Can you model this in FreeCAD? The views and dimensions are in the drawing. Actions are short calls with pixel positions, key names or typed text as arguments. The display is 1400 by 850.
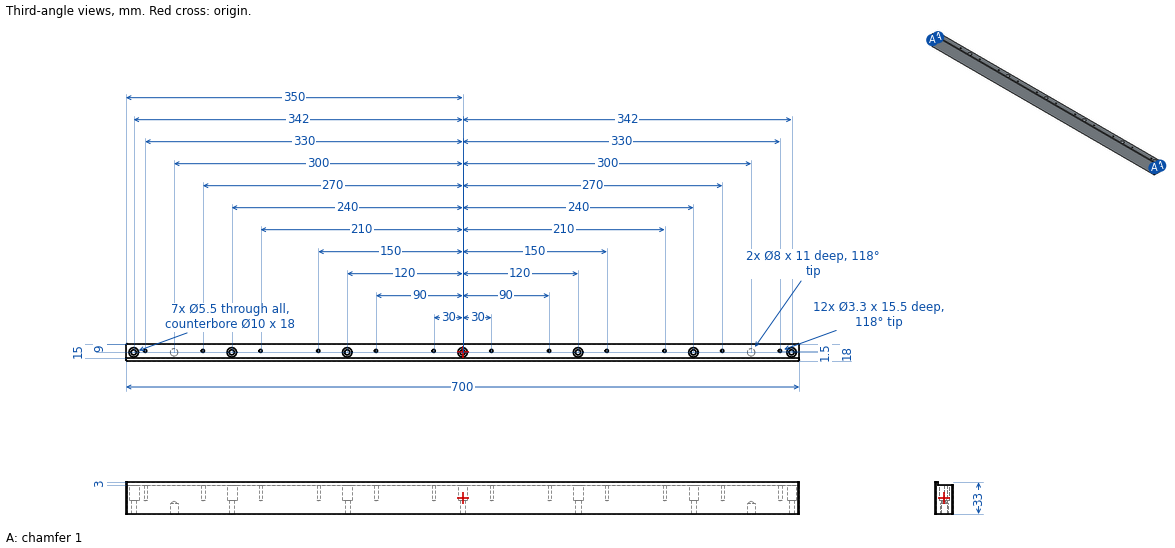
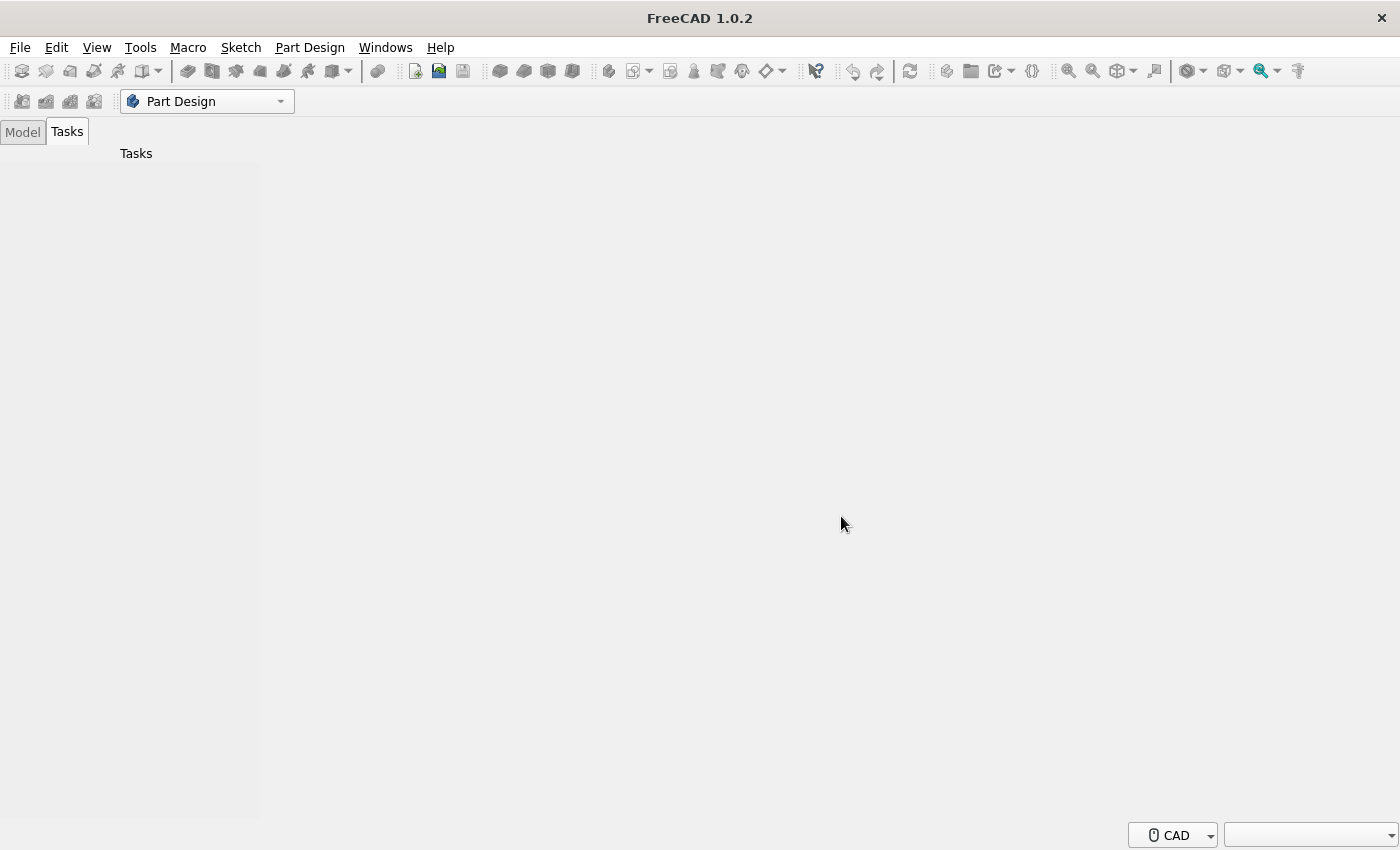
click(416, 72)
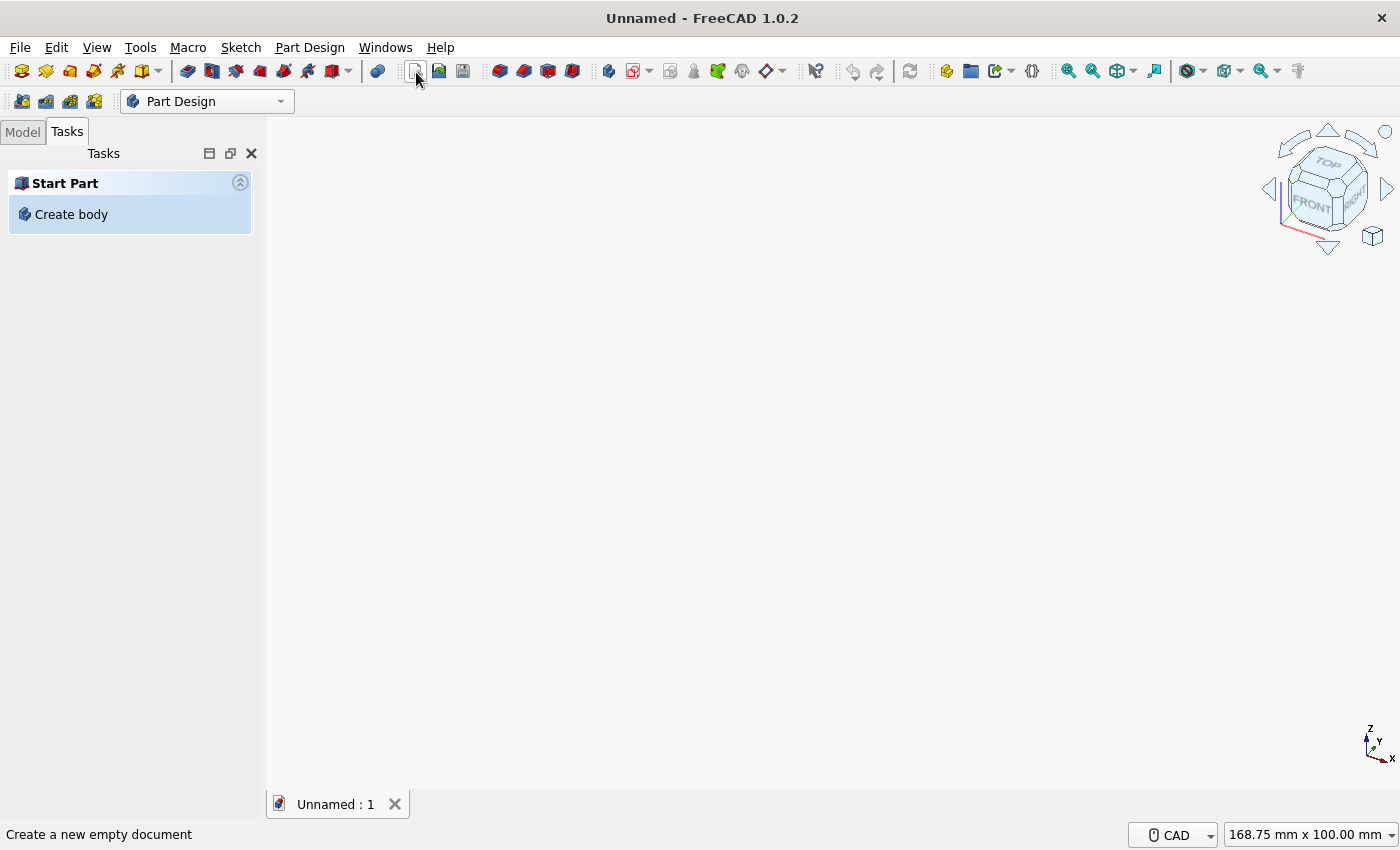
click(634, 72)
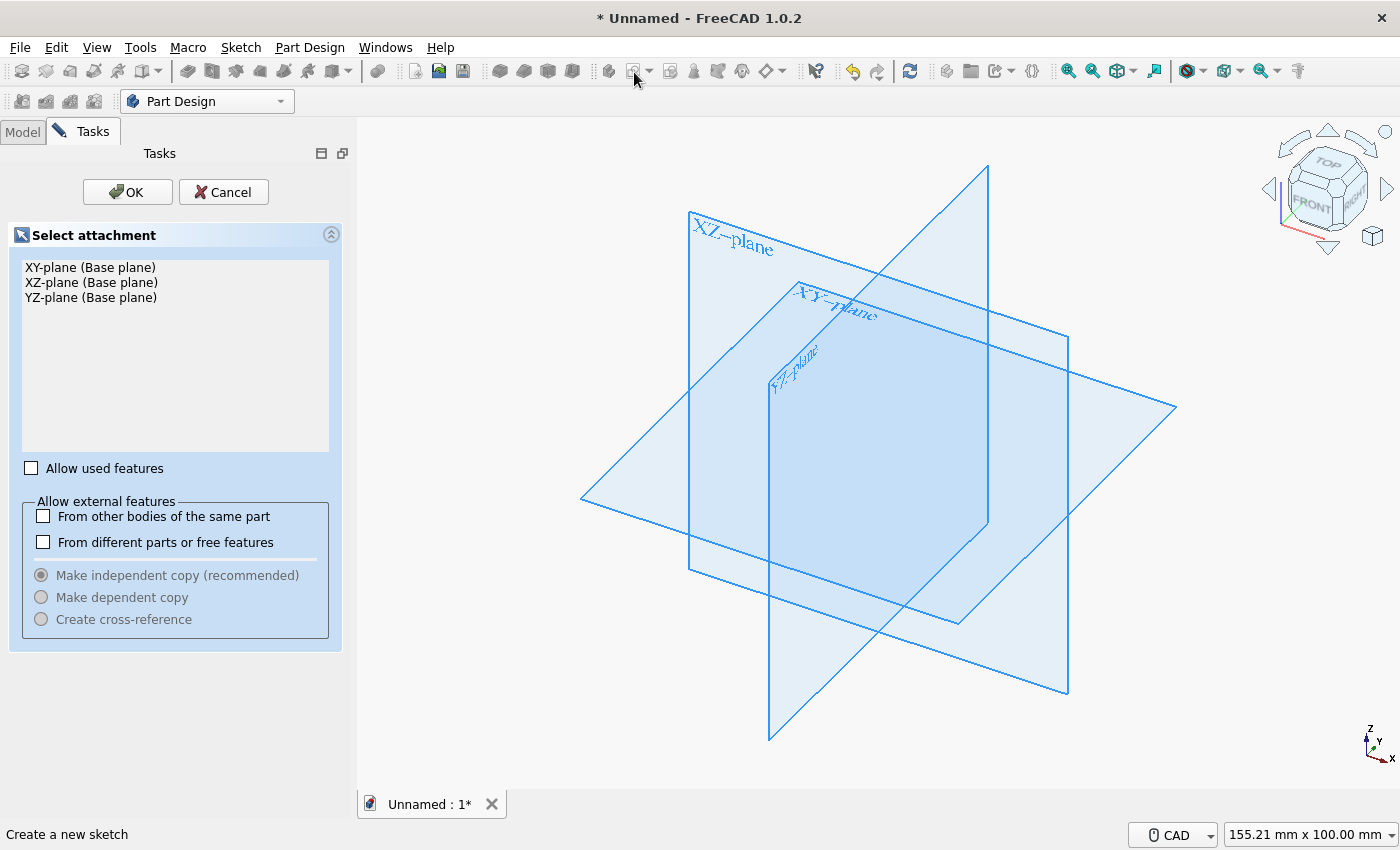
click(82, 268)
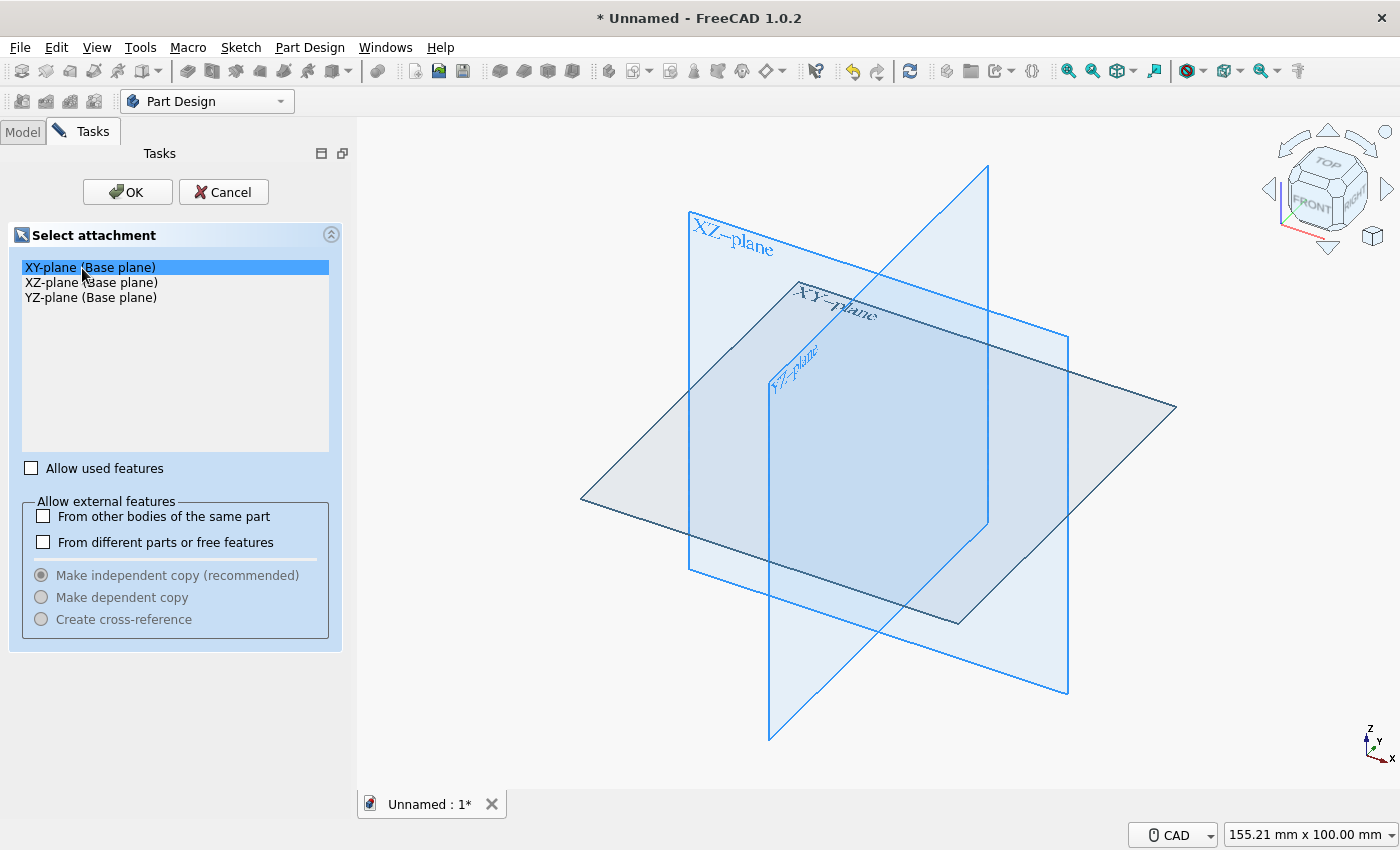
click(128, 192)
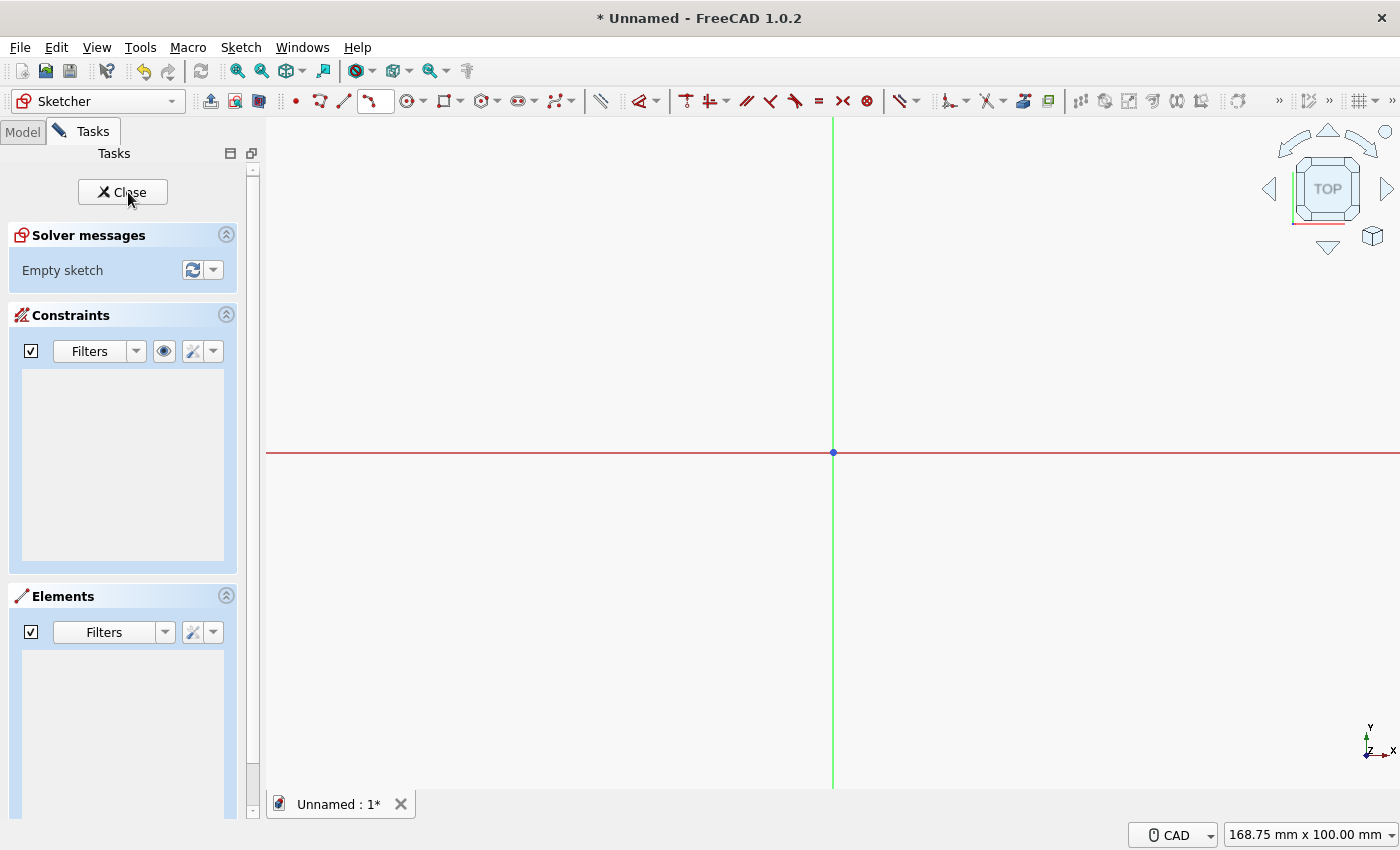
scroll(754, 453, down, 10)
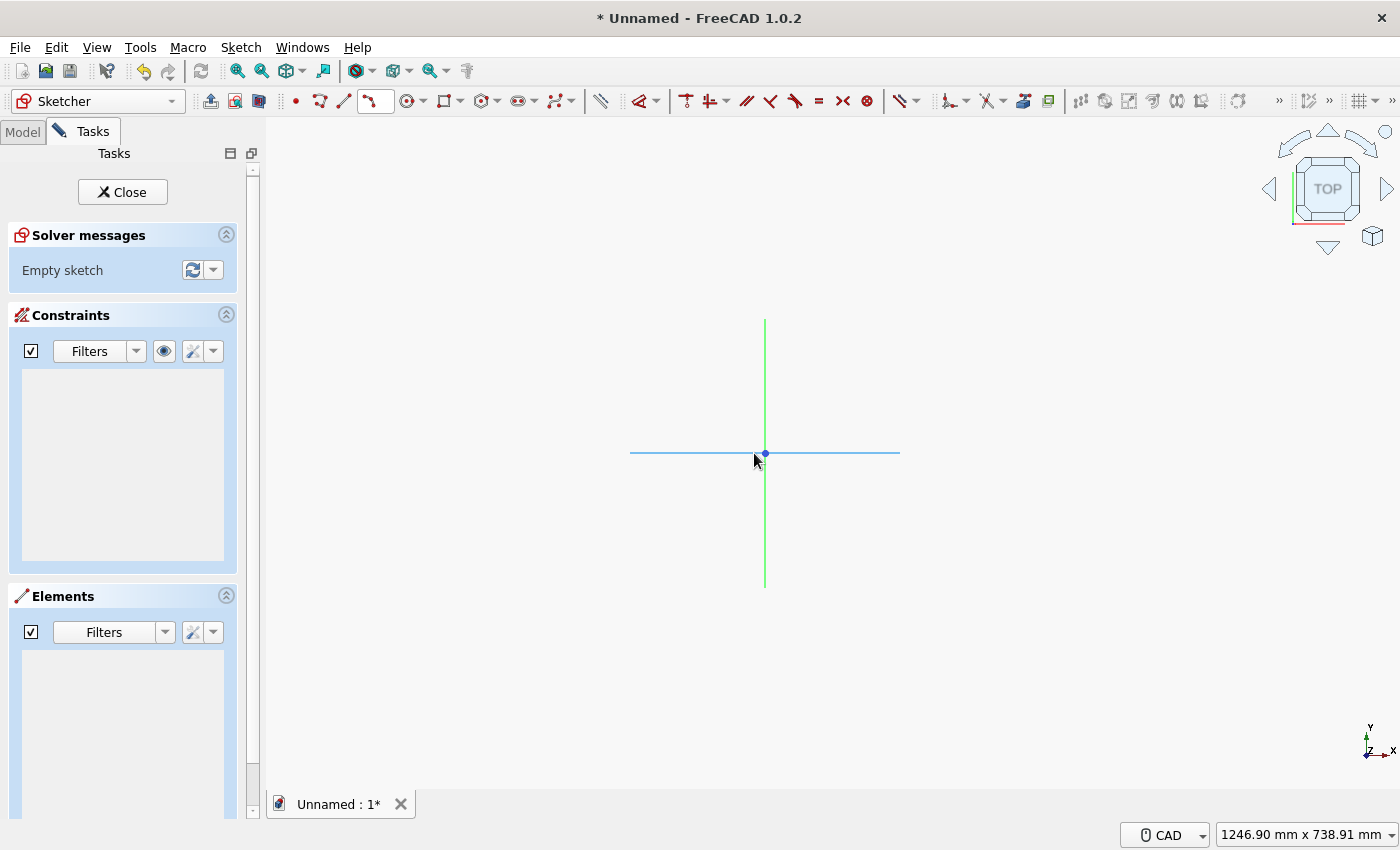
click(462, 102)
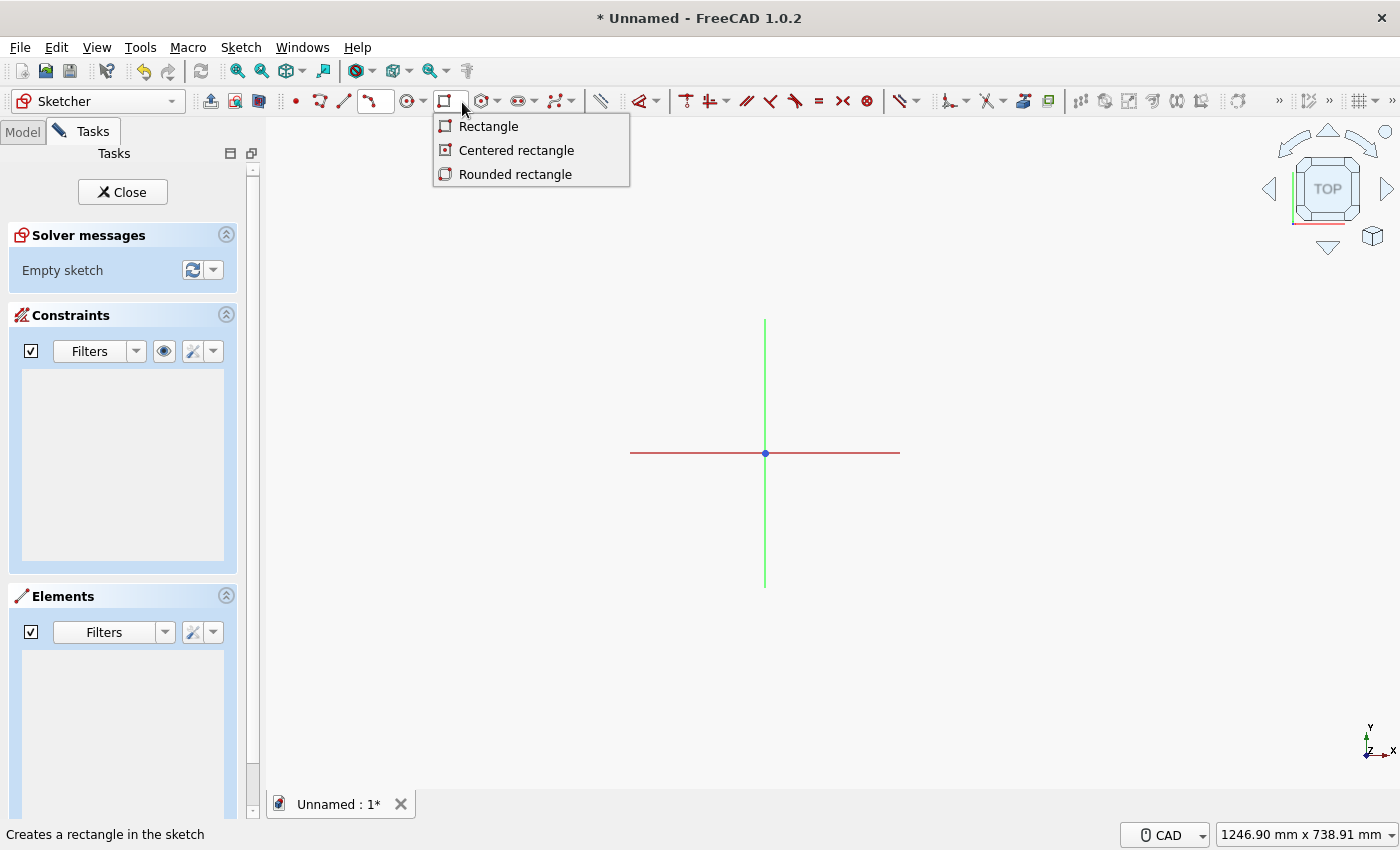
click(532, 150)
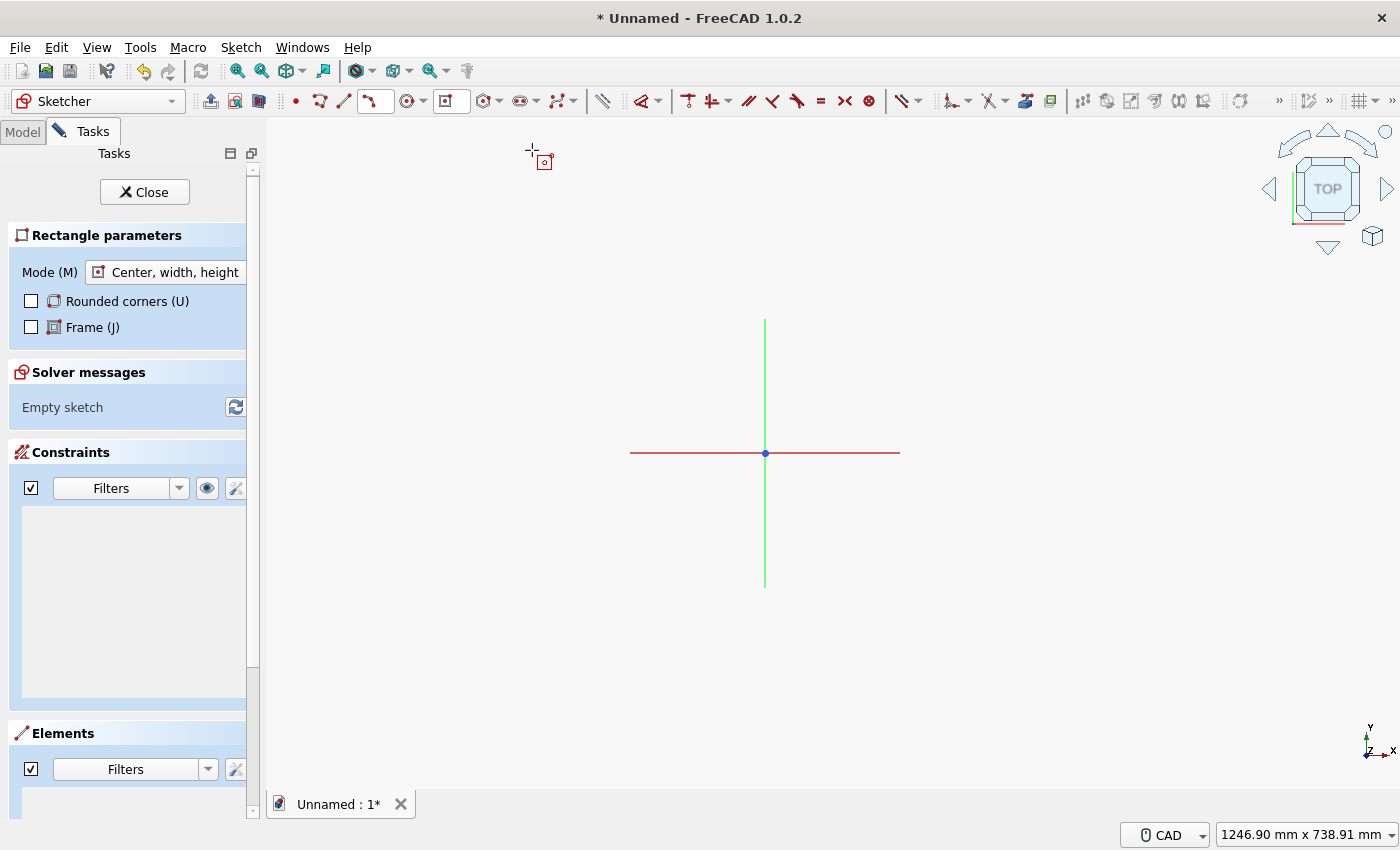
scroll(765, 453, up, 4)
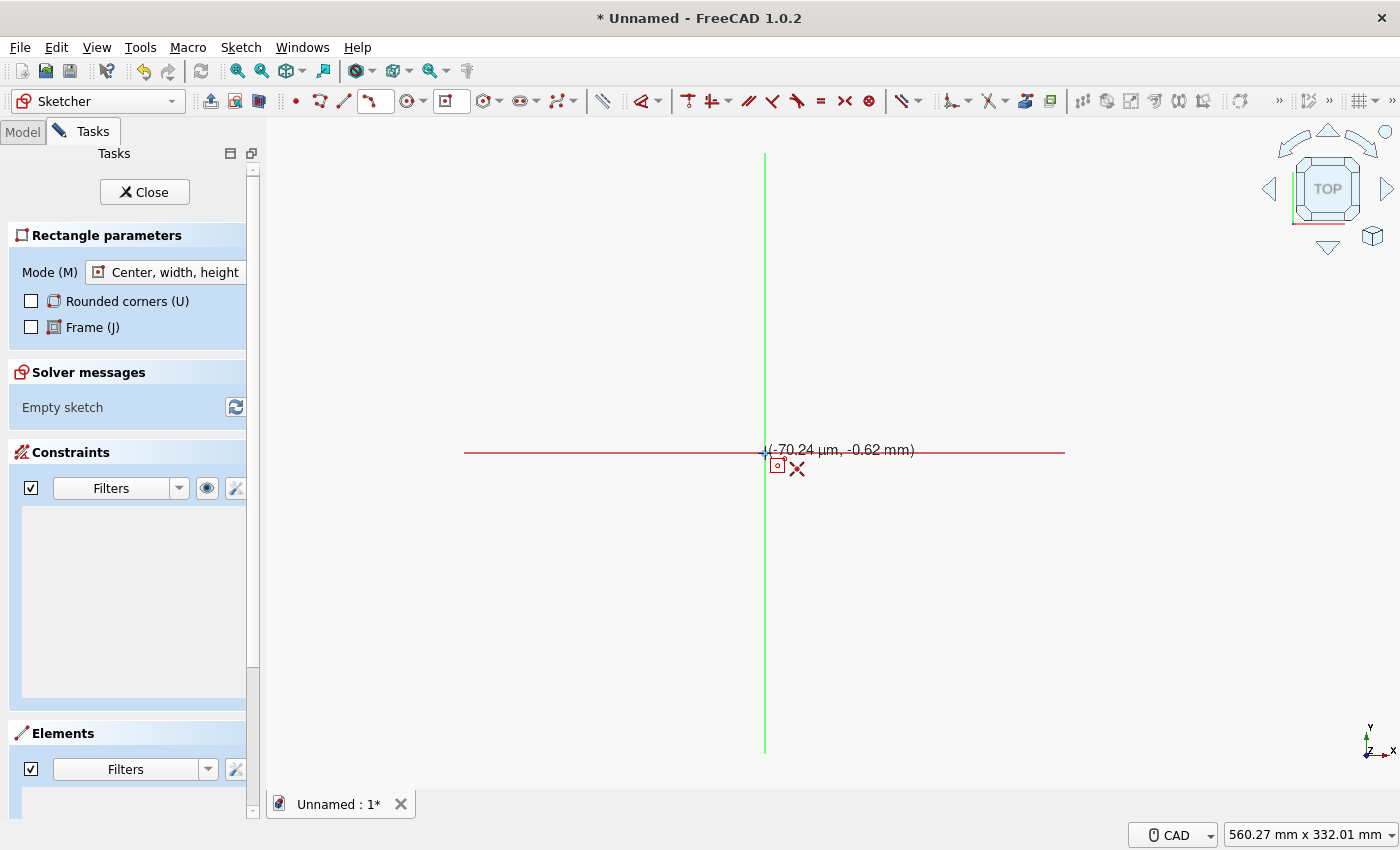
click(765, 453)